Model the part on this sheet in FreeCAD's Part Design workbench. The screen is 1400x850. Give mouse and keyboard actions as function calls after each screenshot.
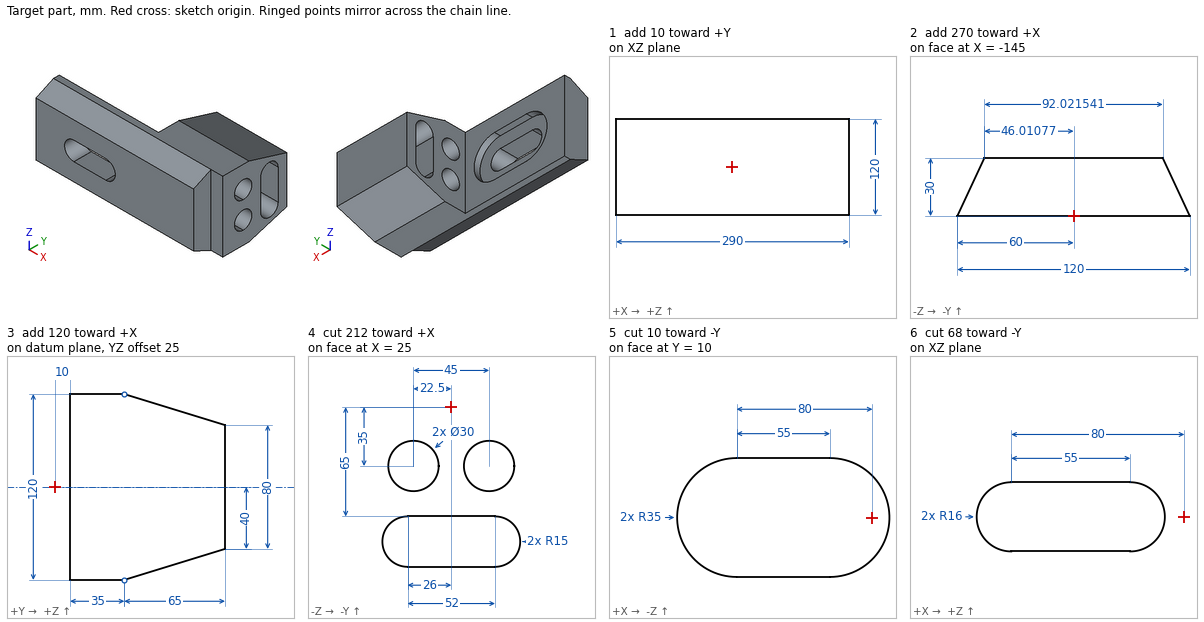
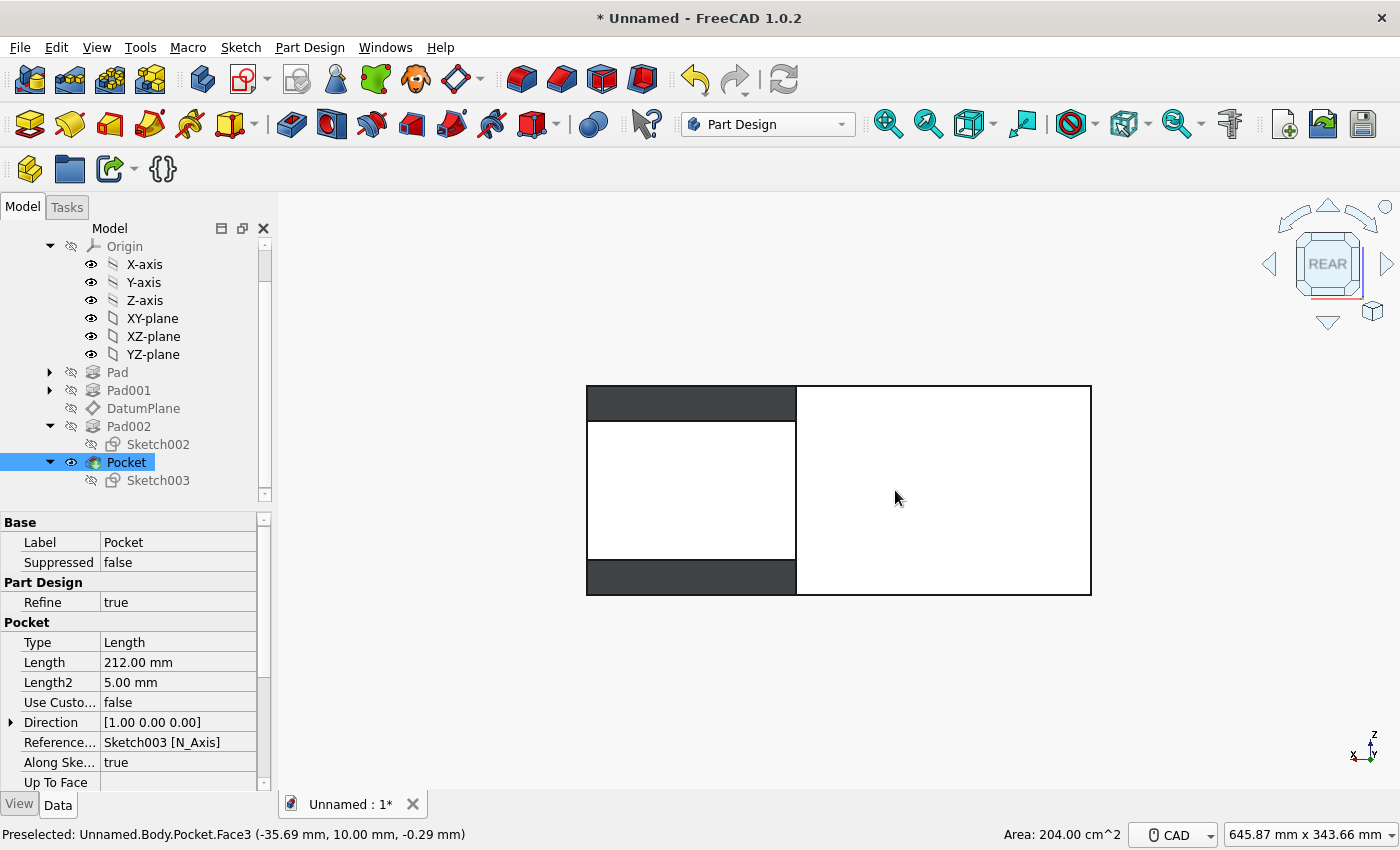
click(244, 80)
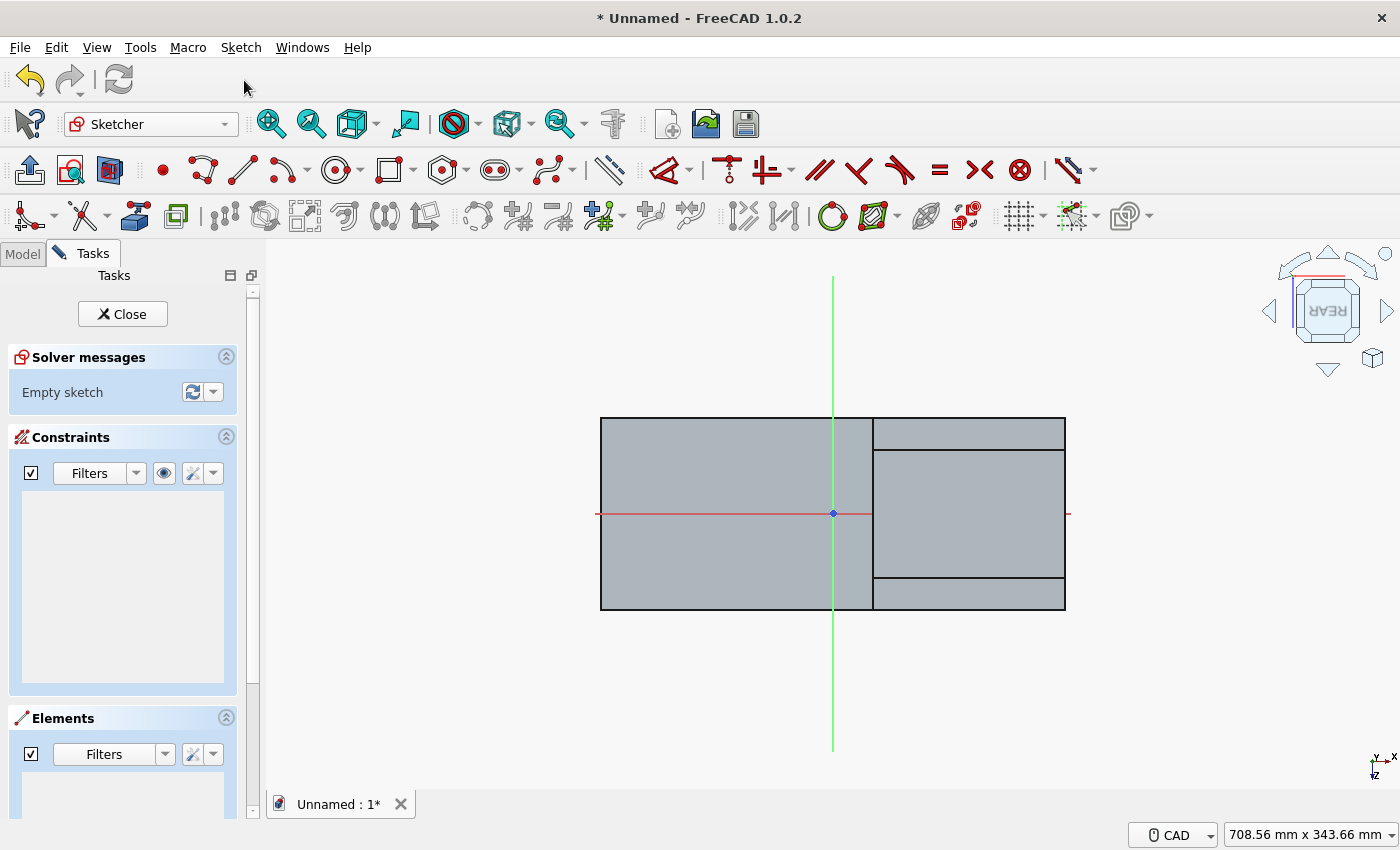
key(q)
key(s)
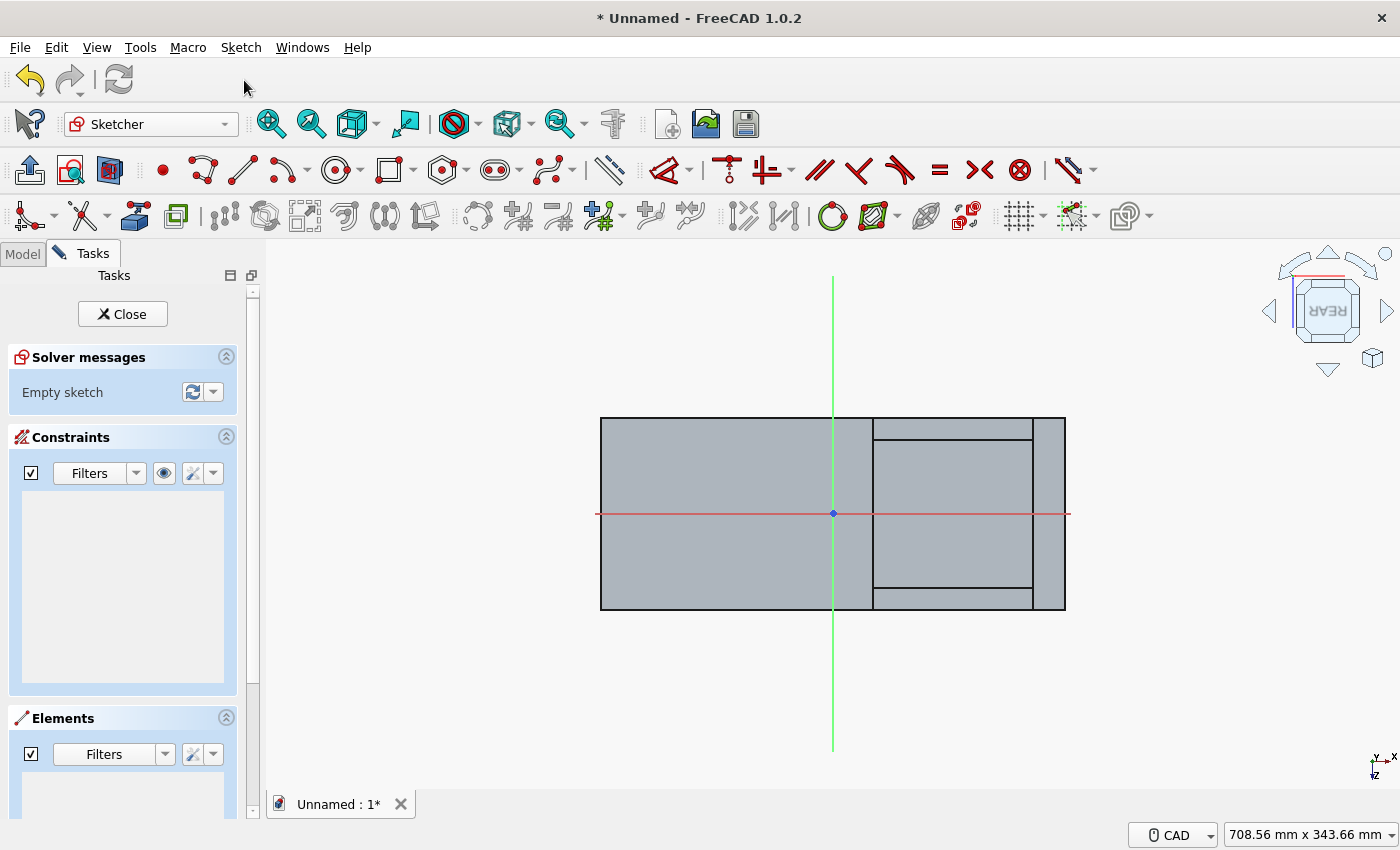
scroll(742, 514, up, 6)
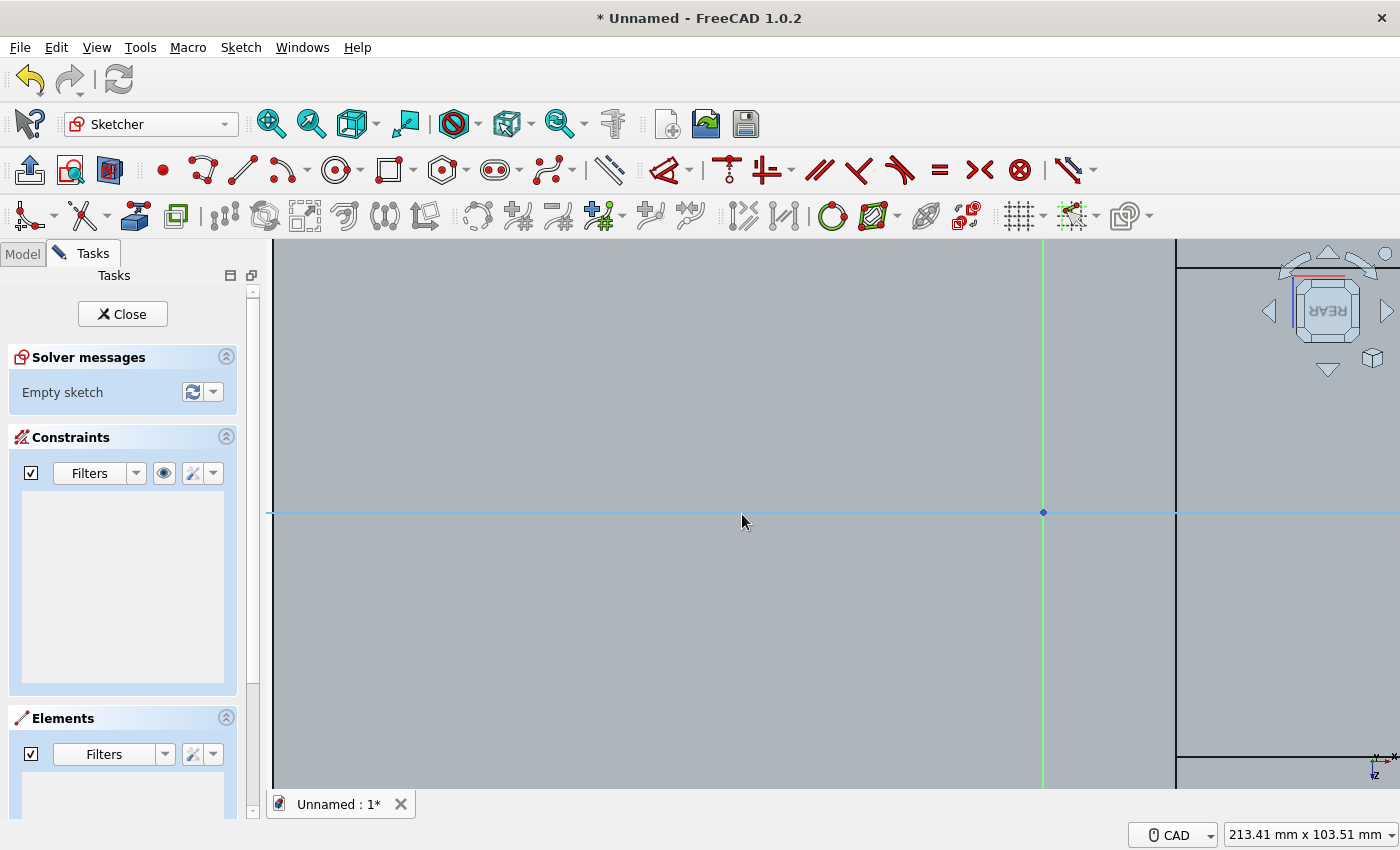
click(496, 170)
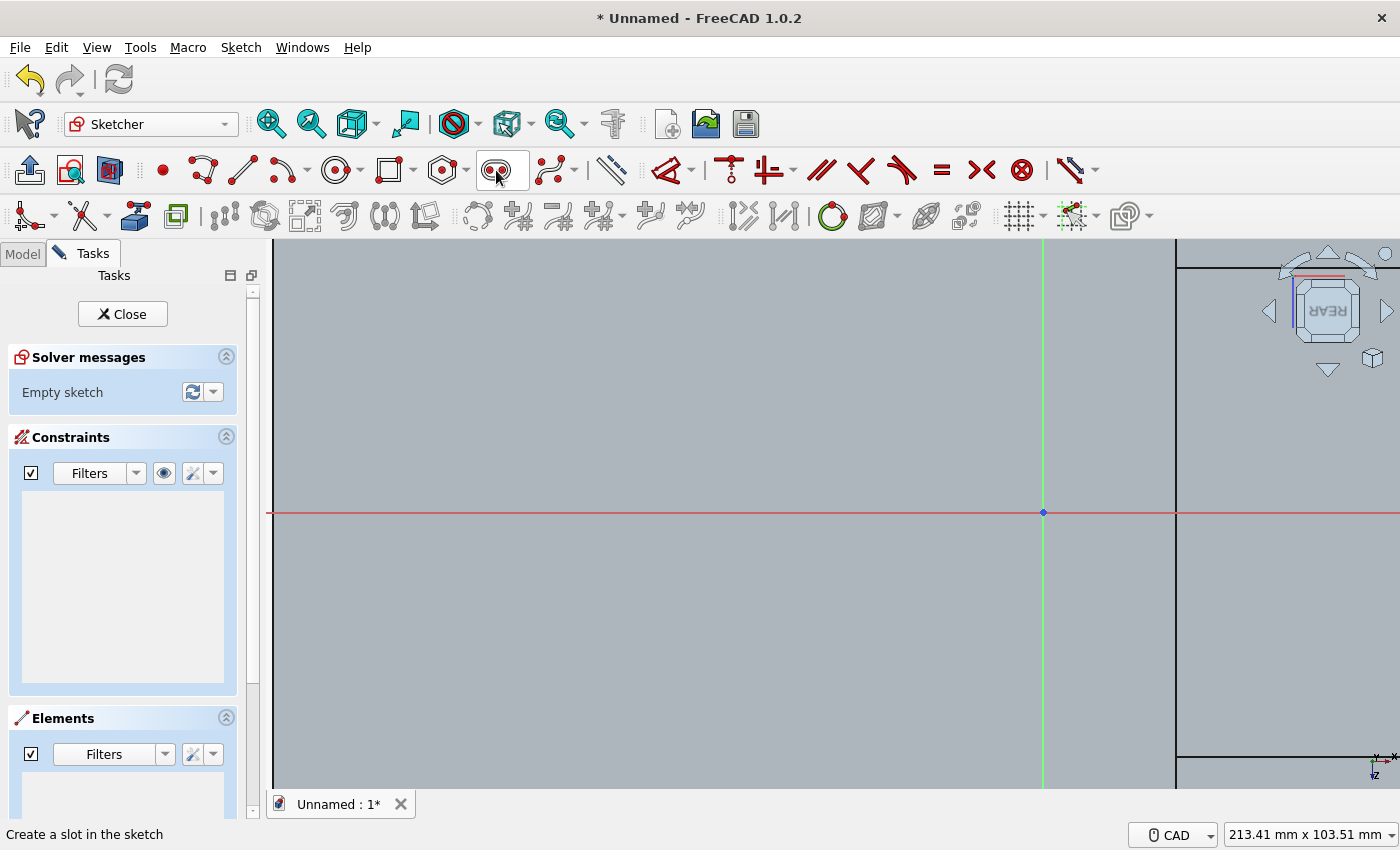
click(618, 513)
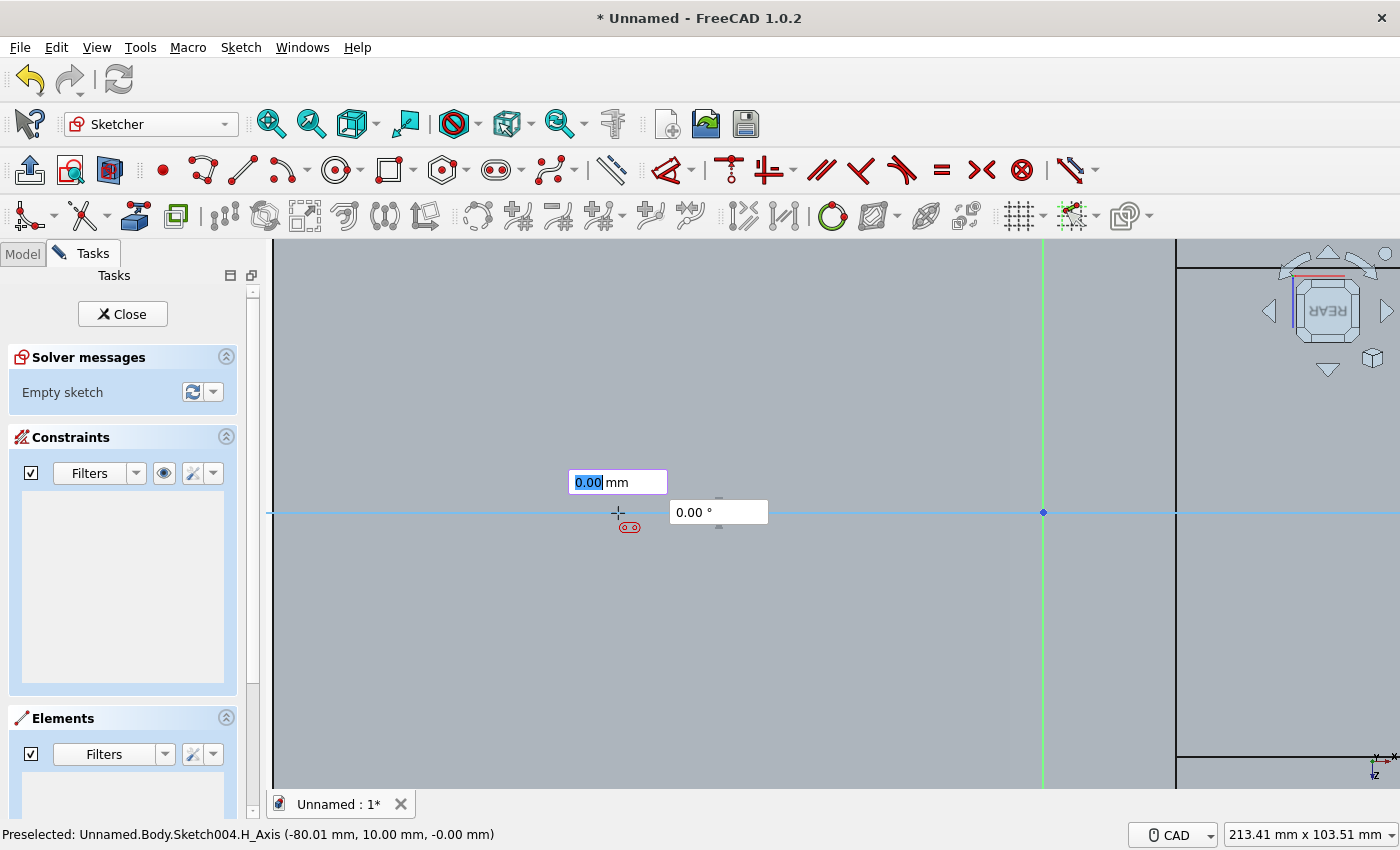
click(910, 504)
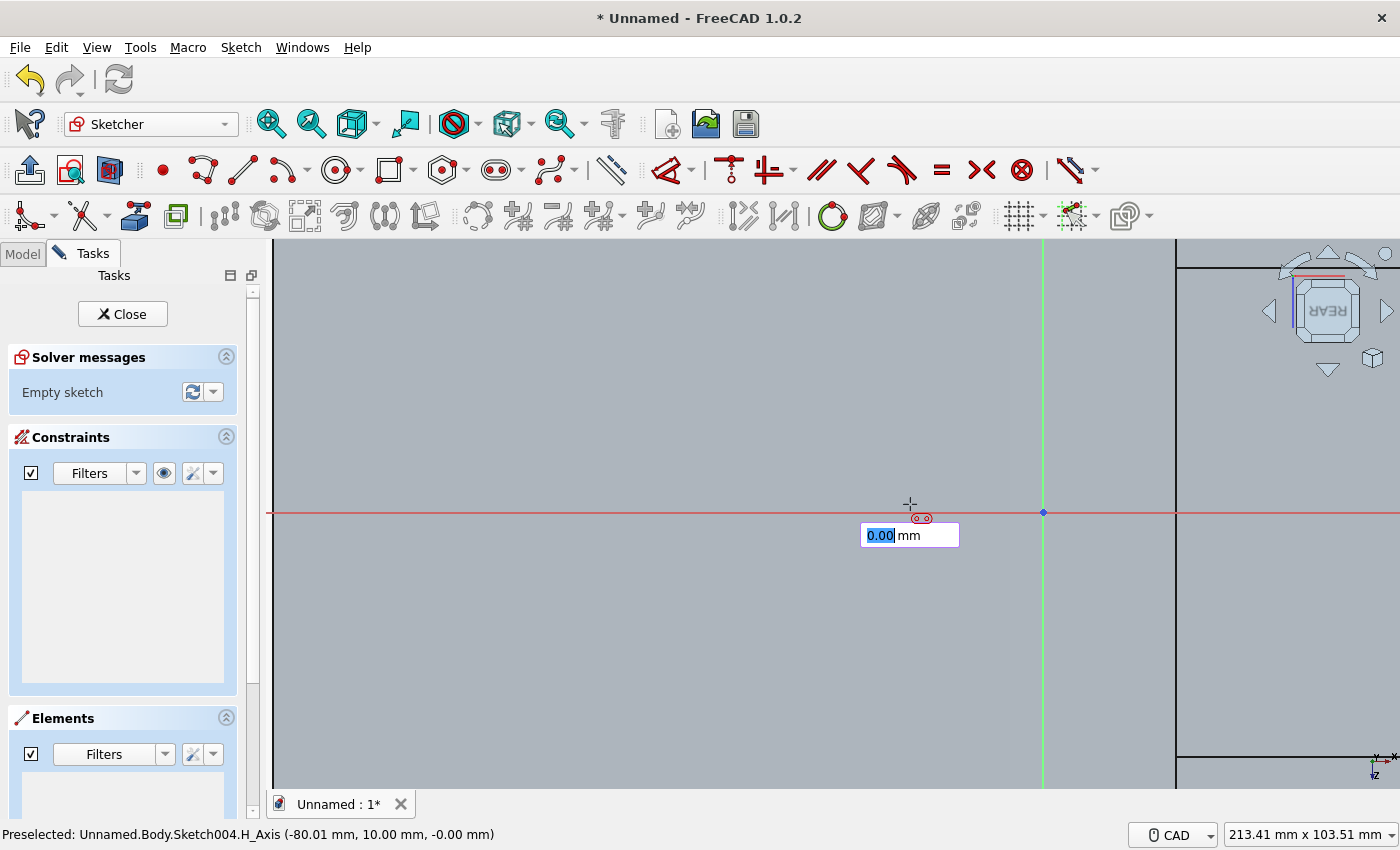
click(764, 327)
key(Escape)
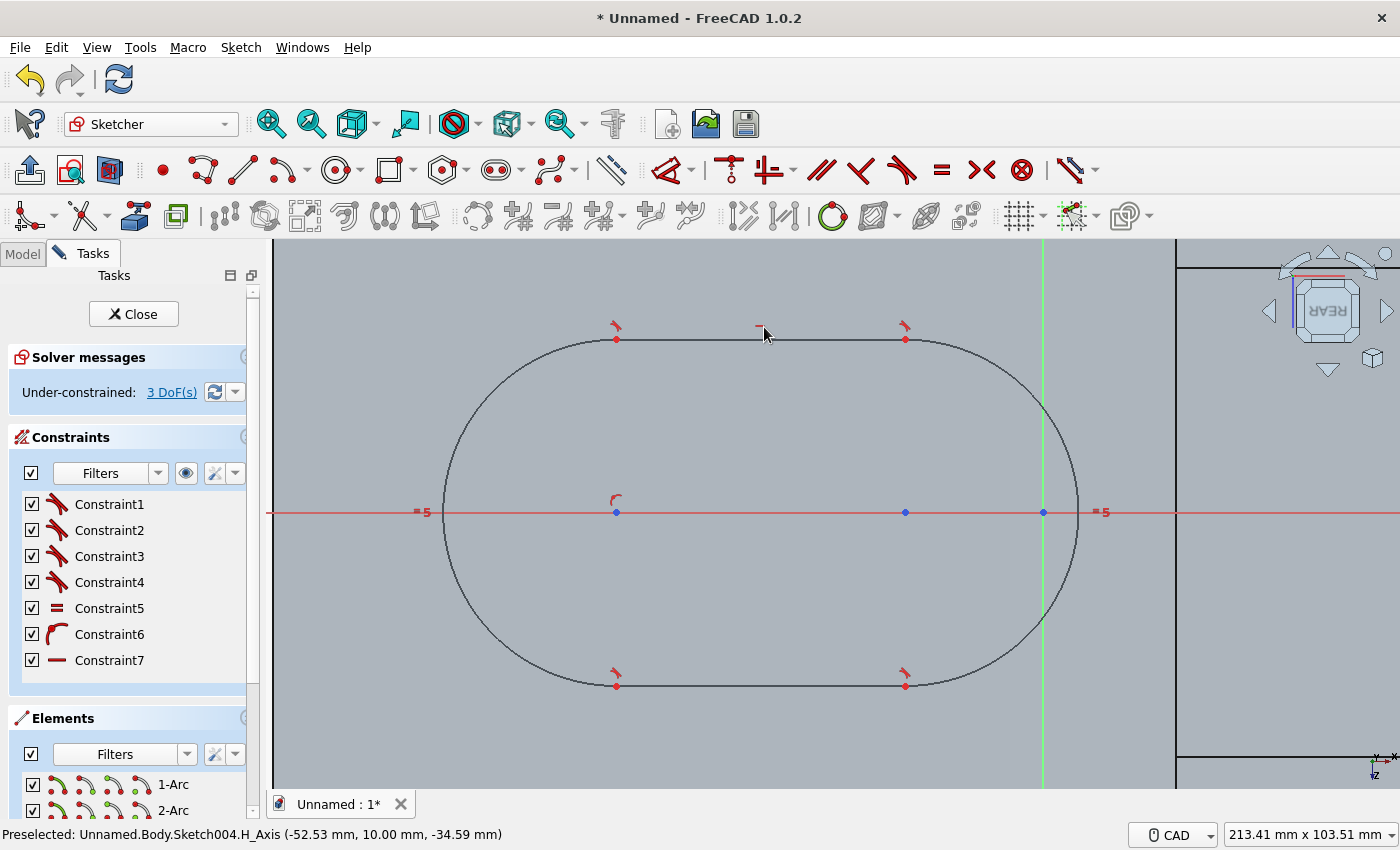
key(d)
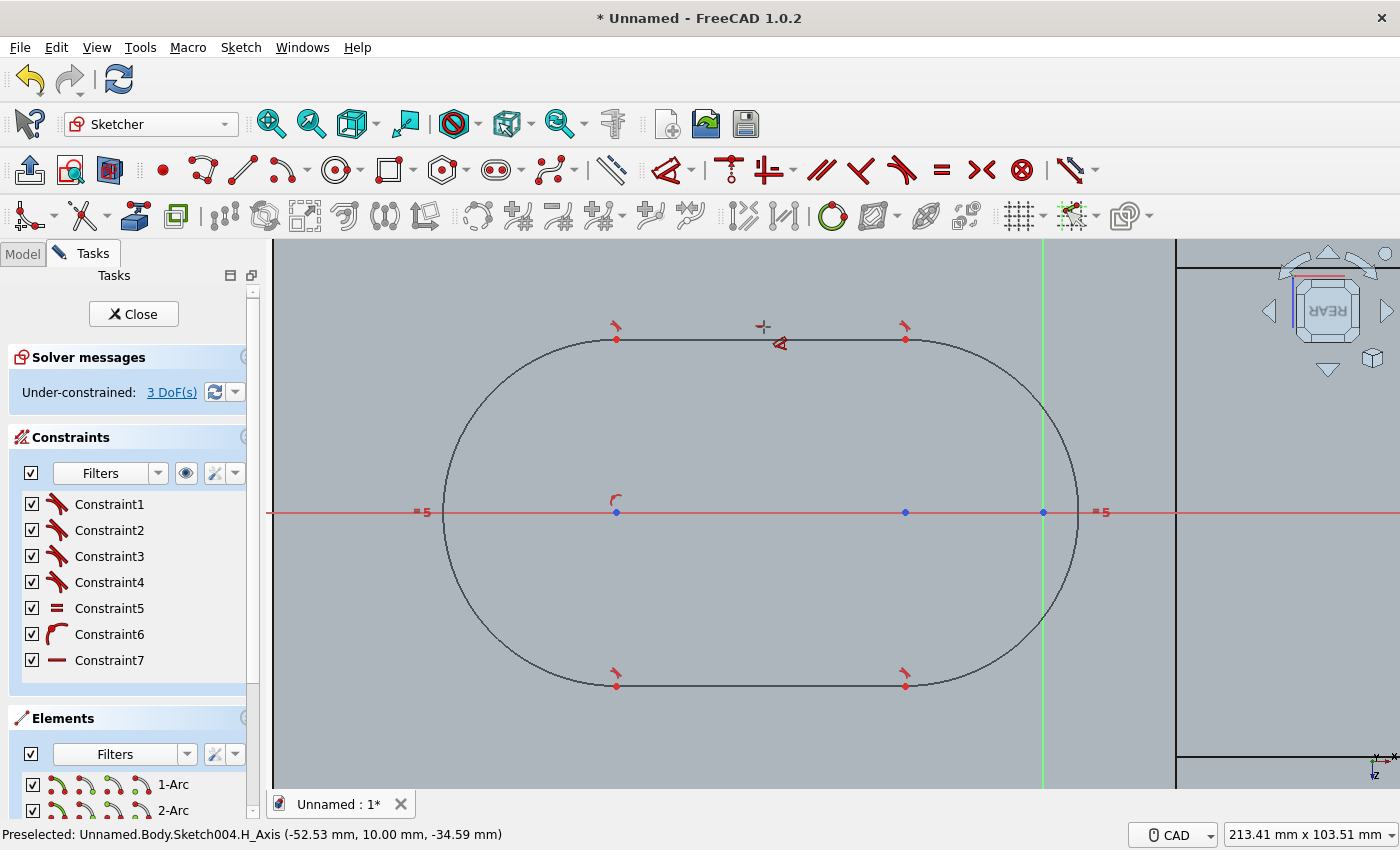
click(476, 411)
click(450, 392)